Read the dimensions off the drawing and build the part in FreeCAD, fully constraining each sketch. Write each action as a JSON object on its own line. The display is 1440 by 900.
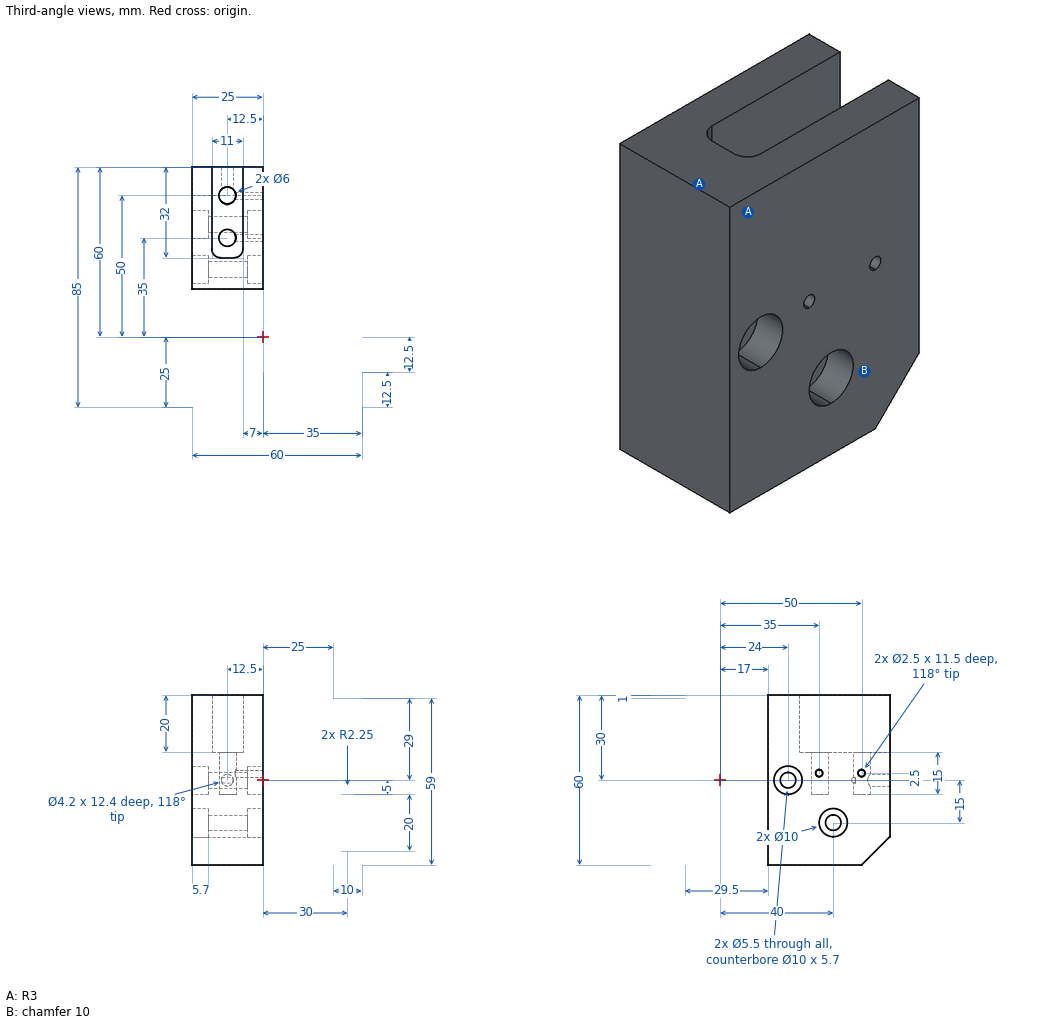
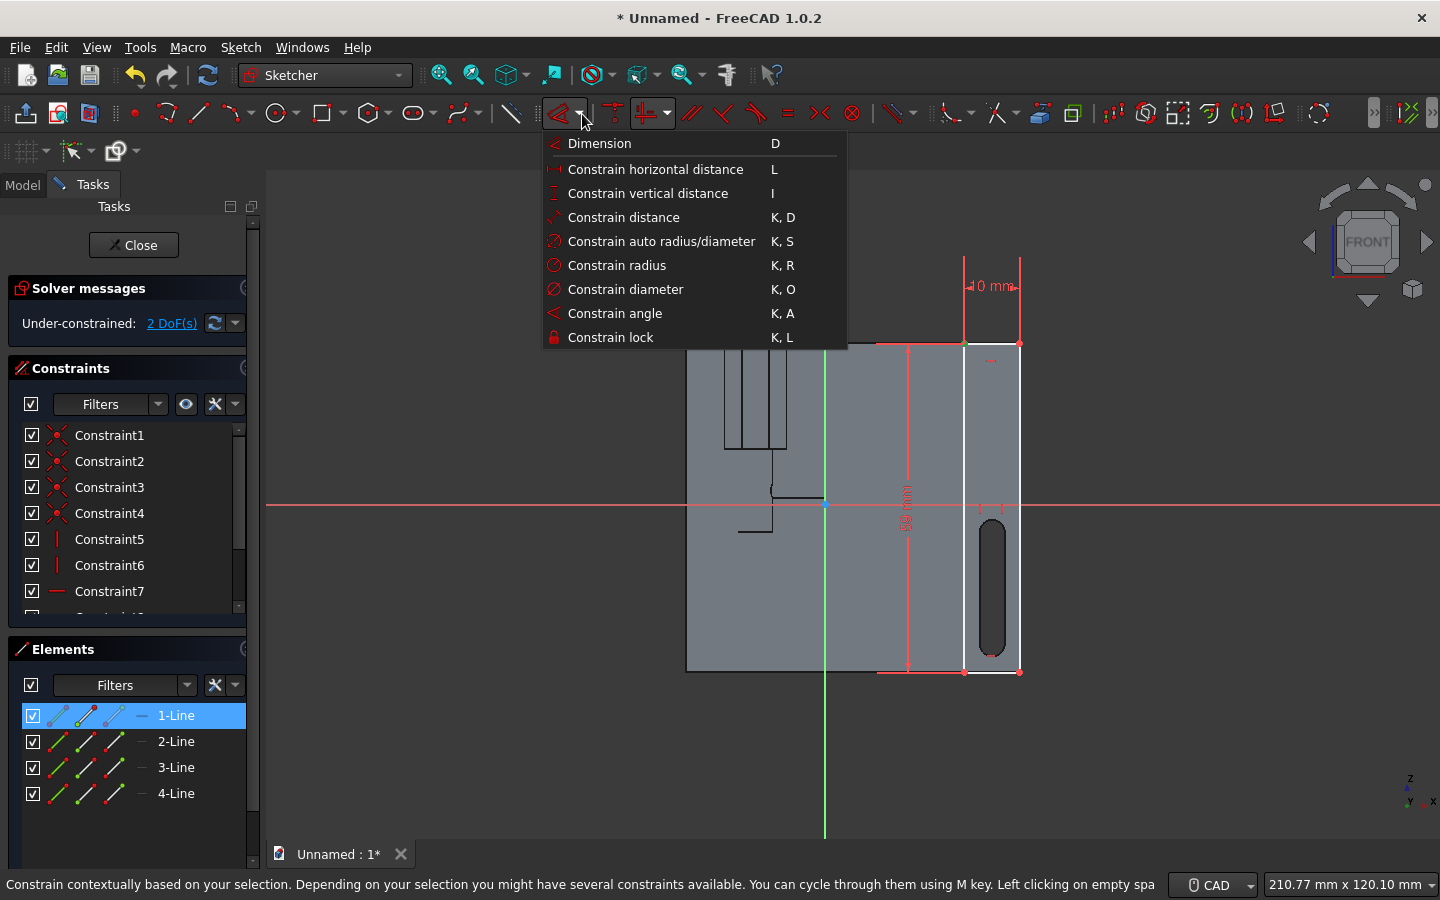
{"action": "left_click", "coordinate": [695, 169]}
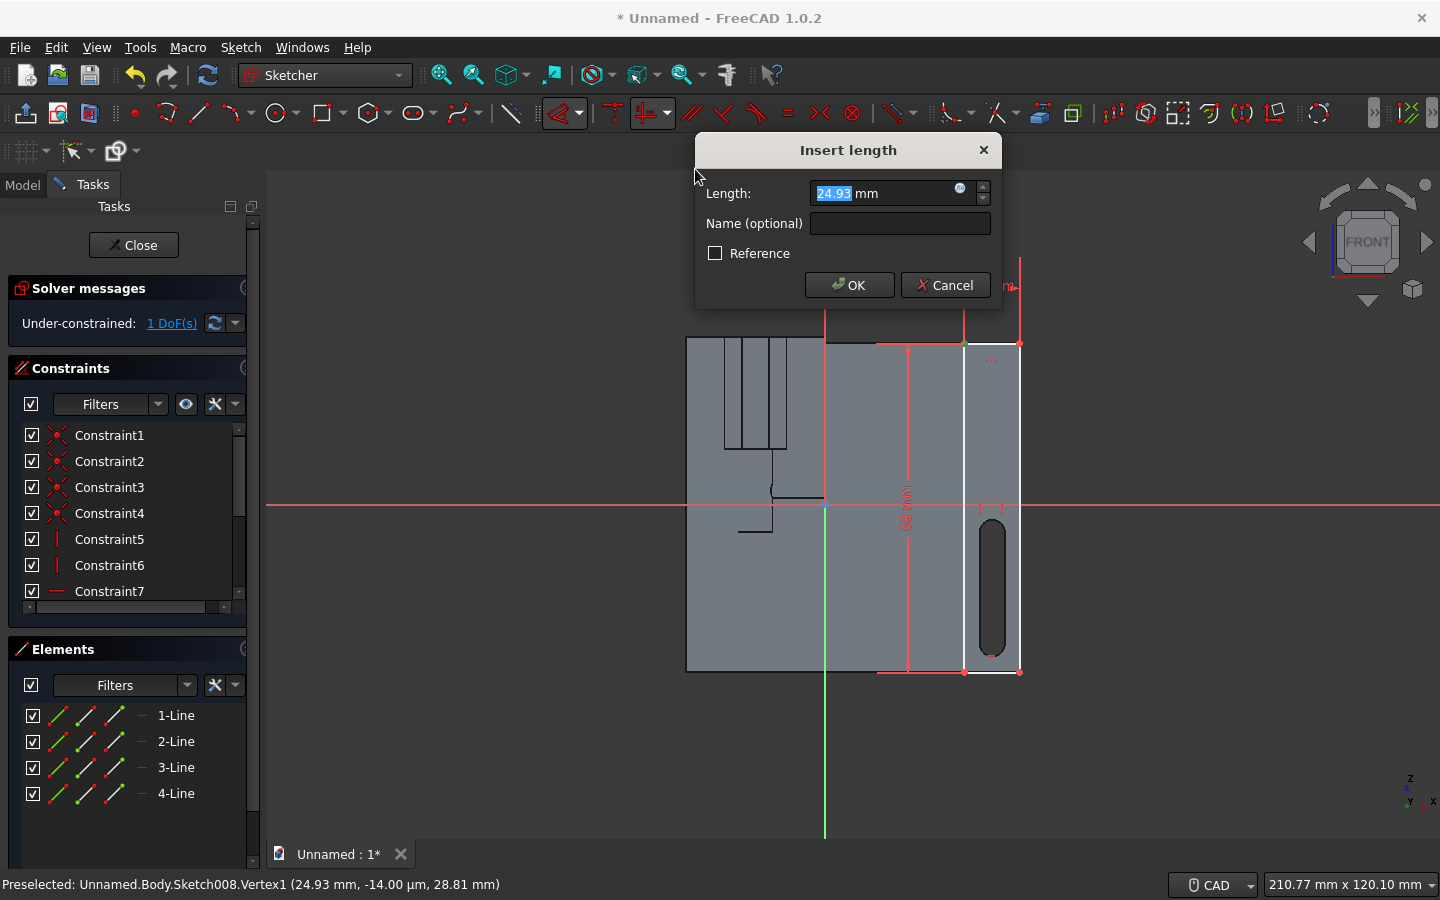
{"action": "type", "text": "25"}
{"action": "key", "text": "Return"}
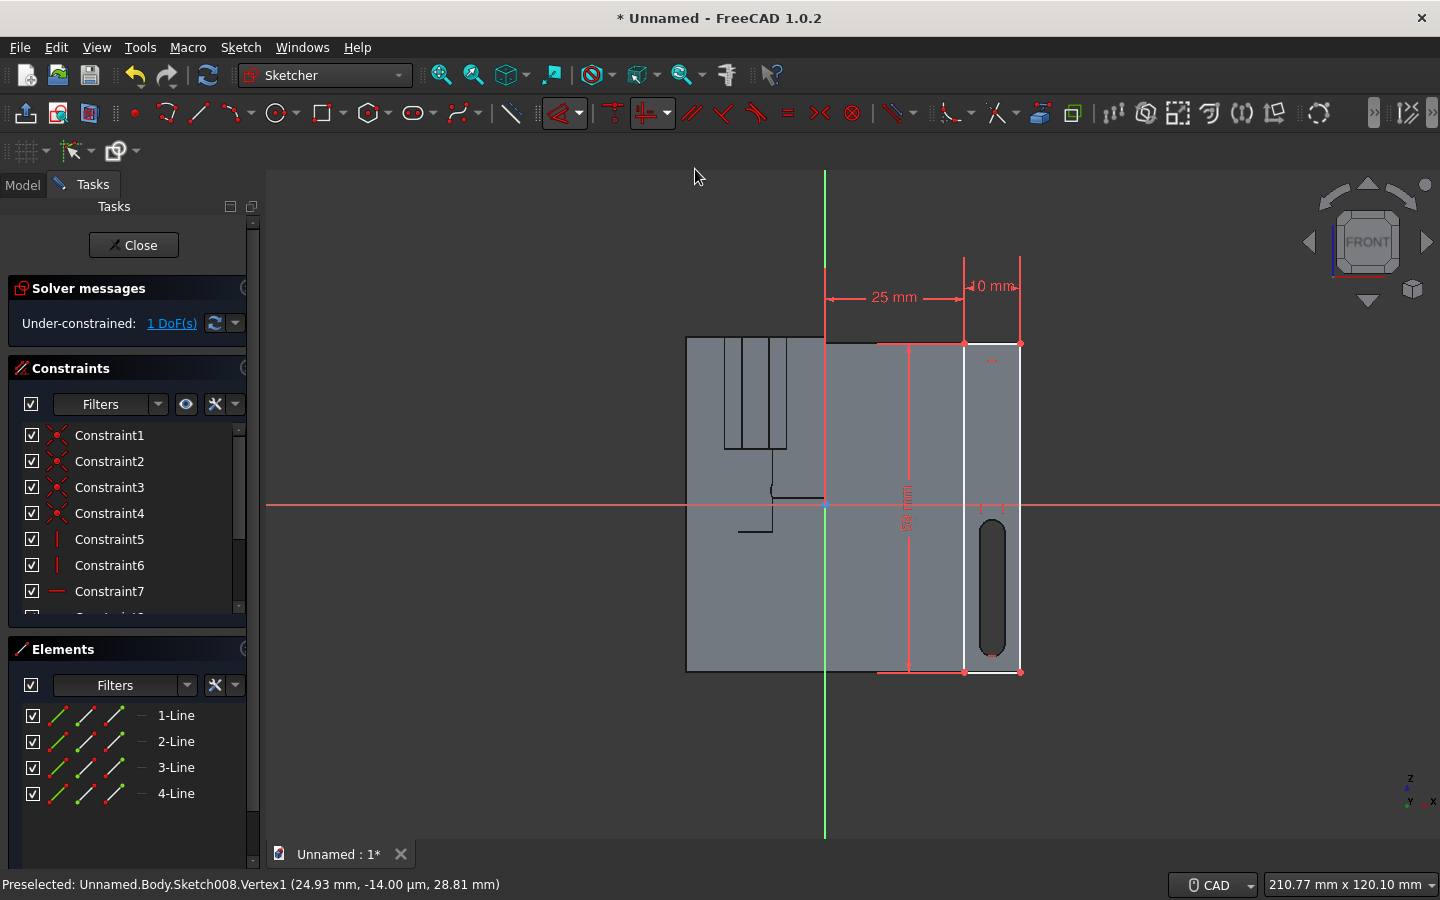
{"action": "left_click", "coordinate": [964, 344]}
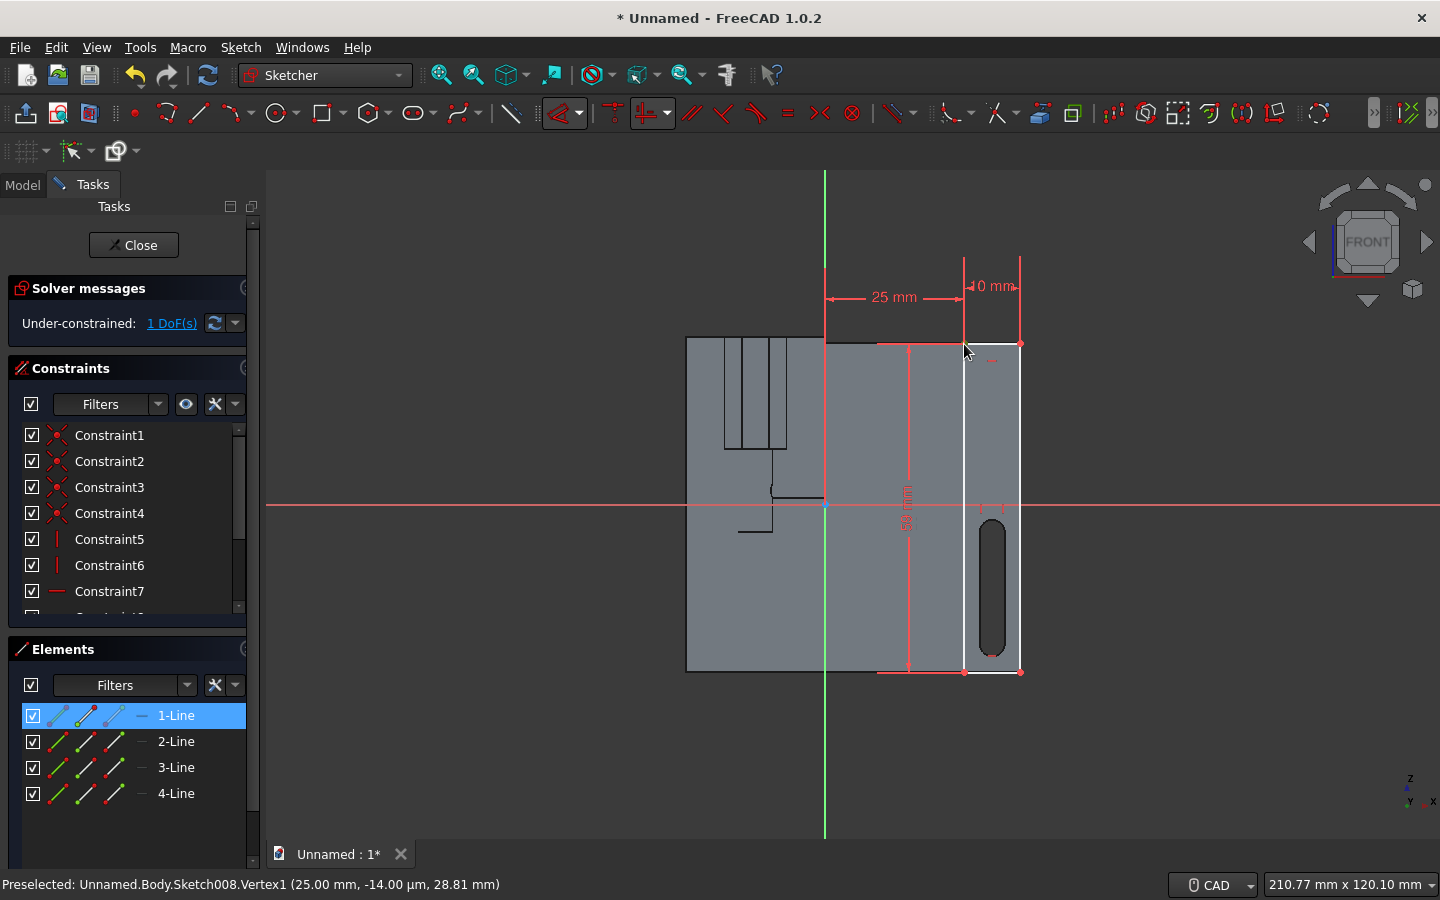
{"action": "key", "text": "i"}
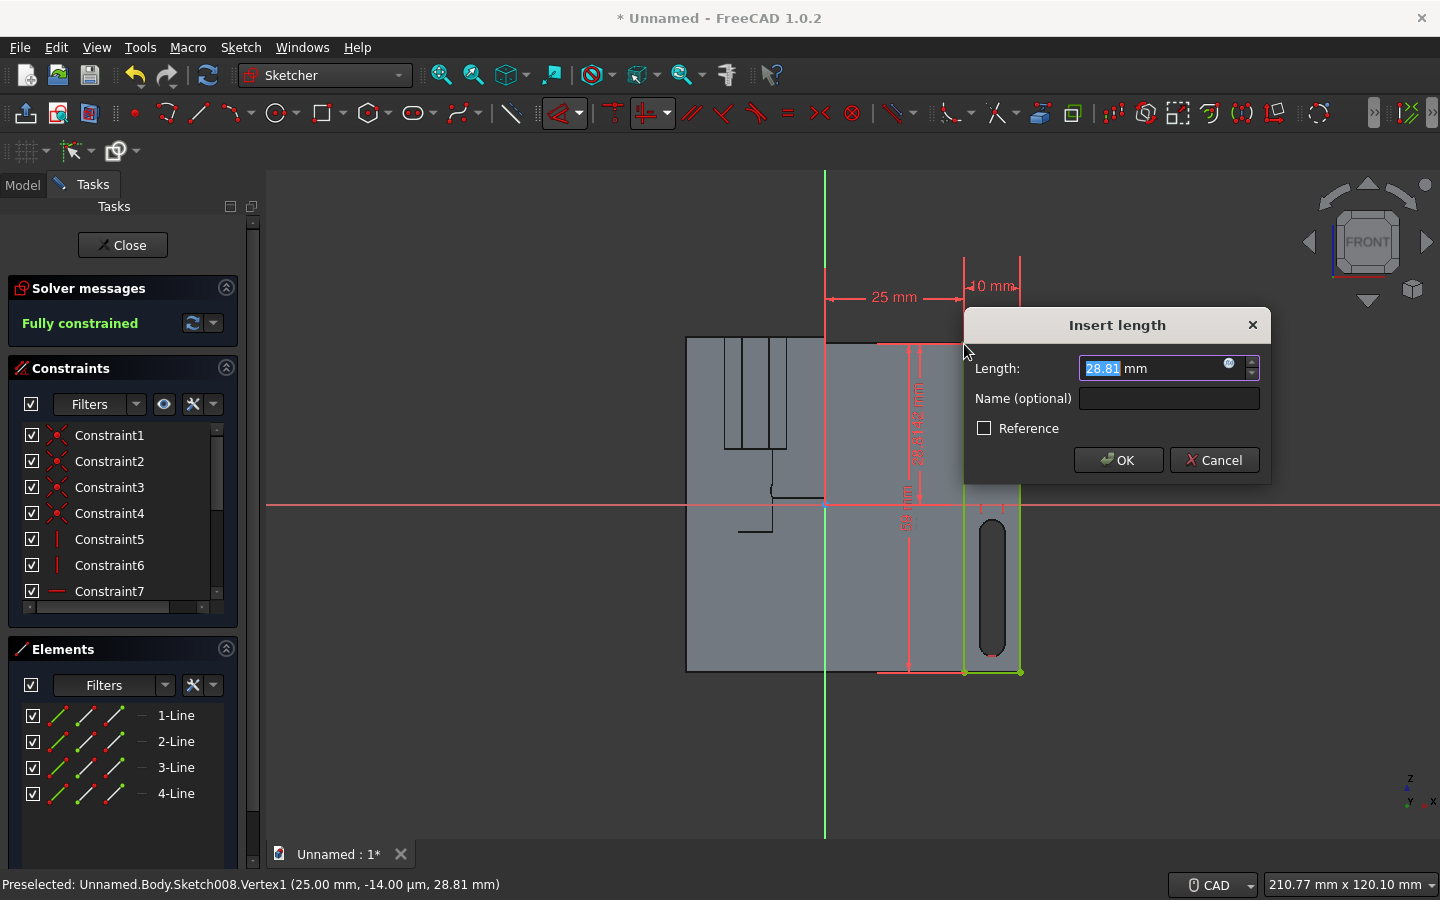
{"action": "type", "text": "29"}
{"action": "key", "text": "Return"}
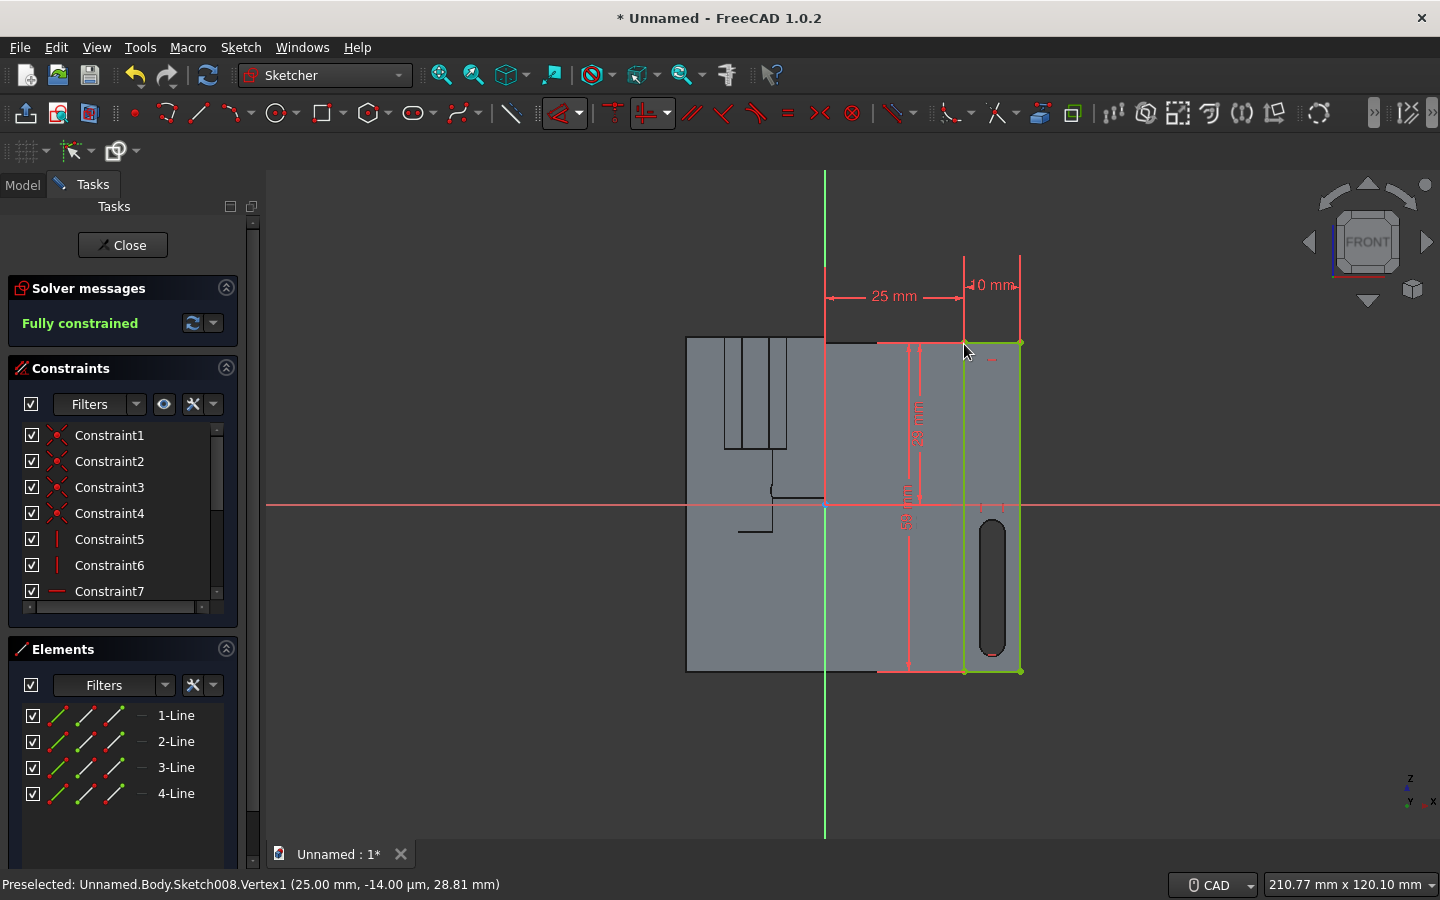
{"action": "left_click", "coordinate": [123, 245]}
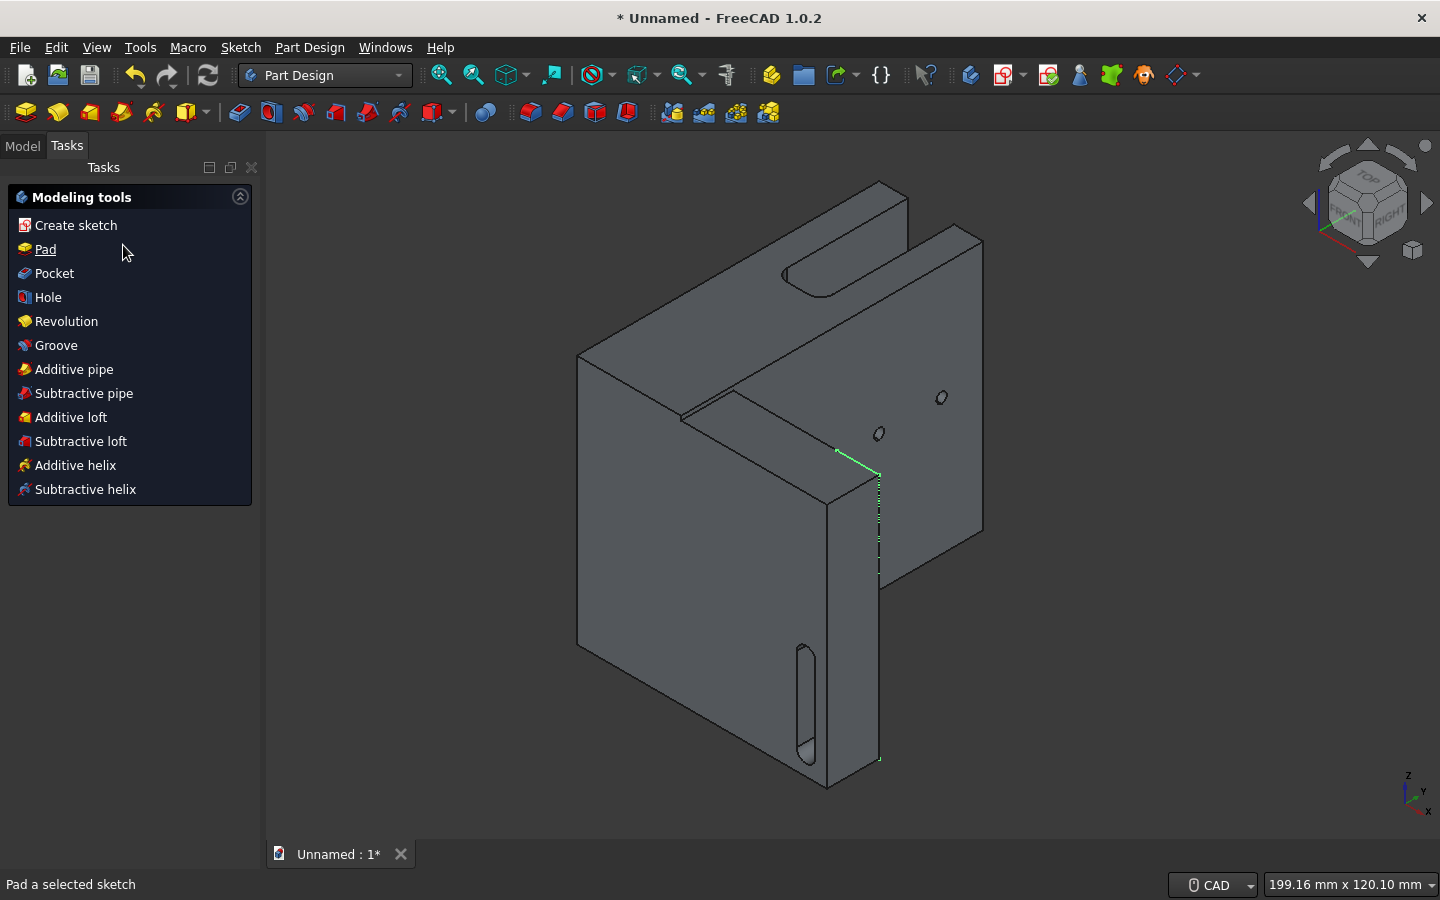
{"action": "left_click", "coordinate": [240, 112]}